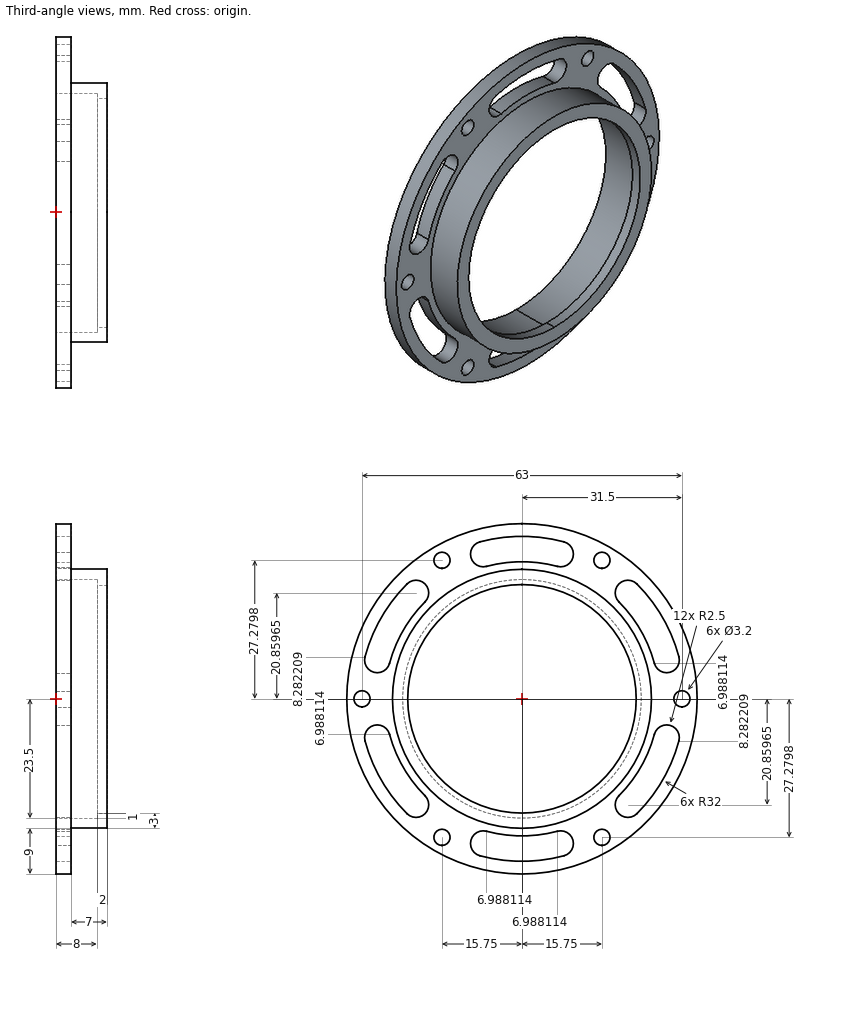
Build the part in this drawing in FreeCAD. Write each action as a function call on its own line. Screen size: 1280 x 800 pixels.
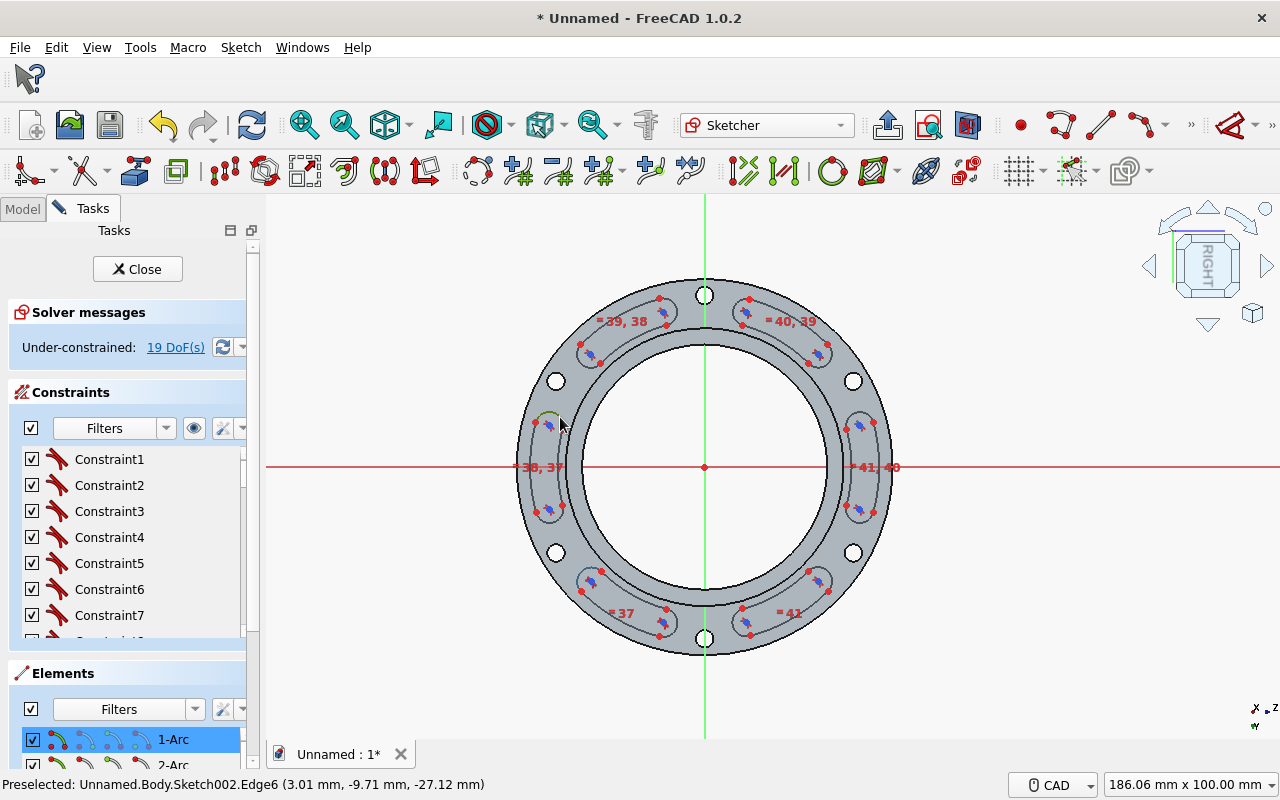
click(676, 317)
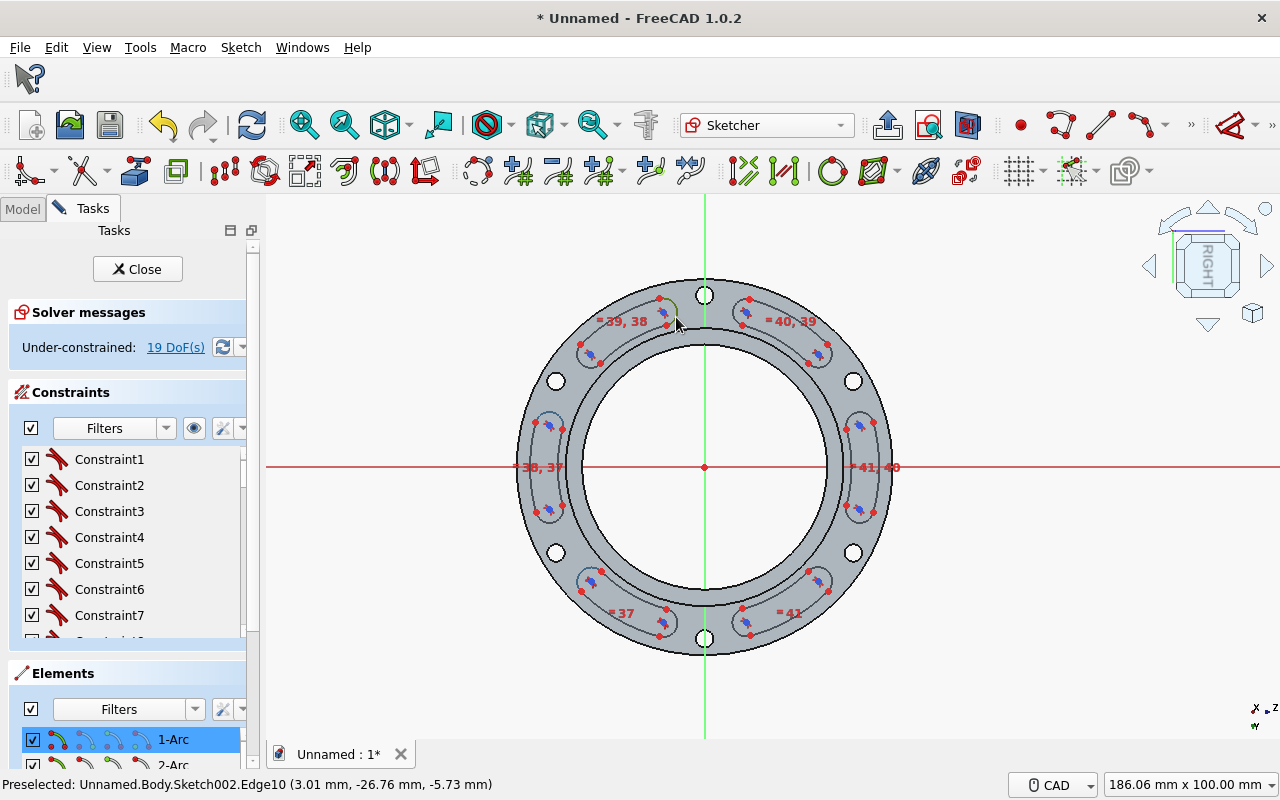
click(820, 367)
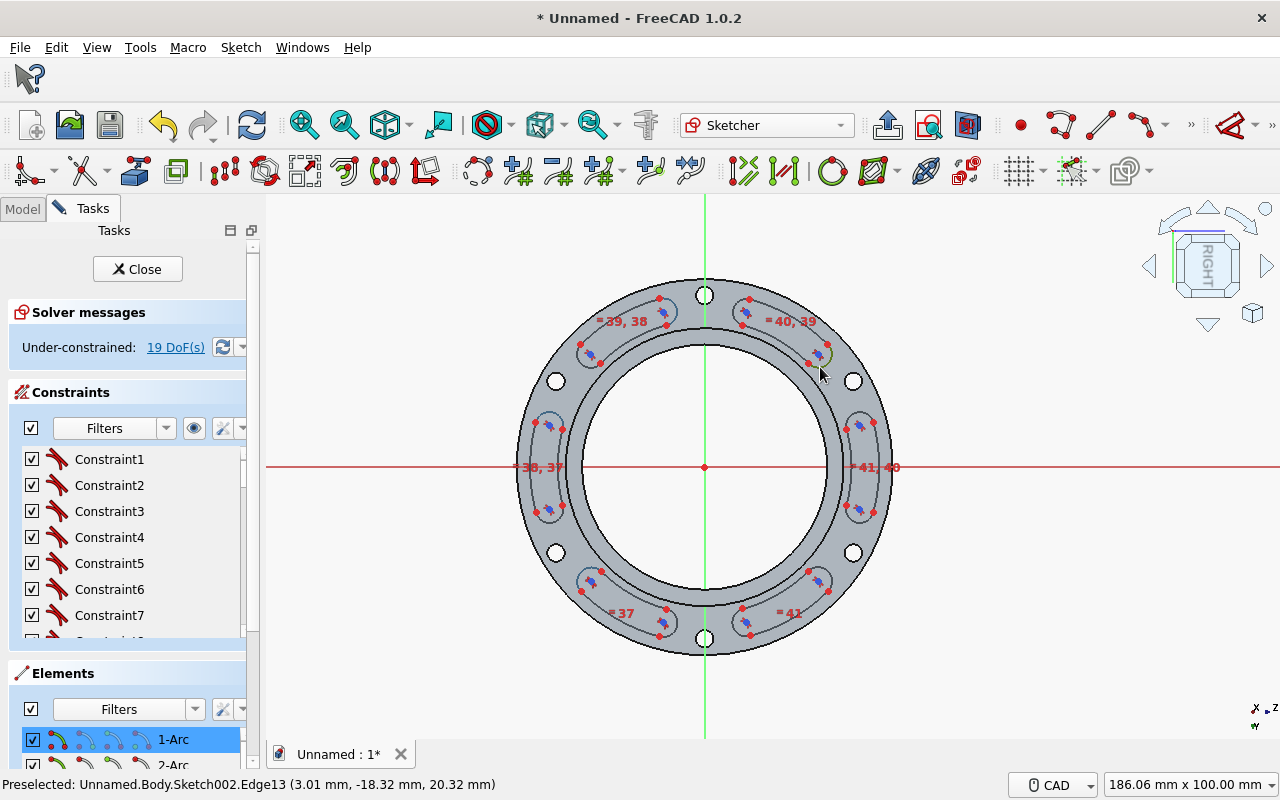
click(849, 518)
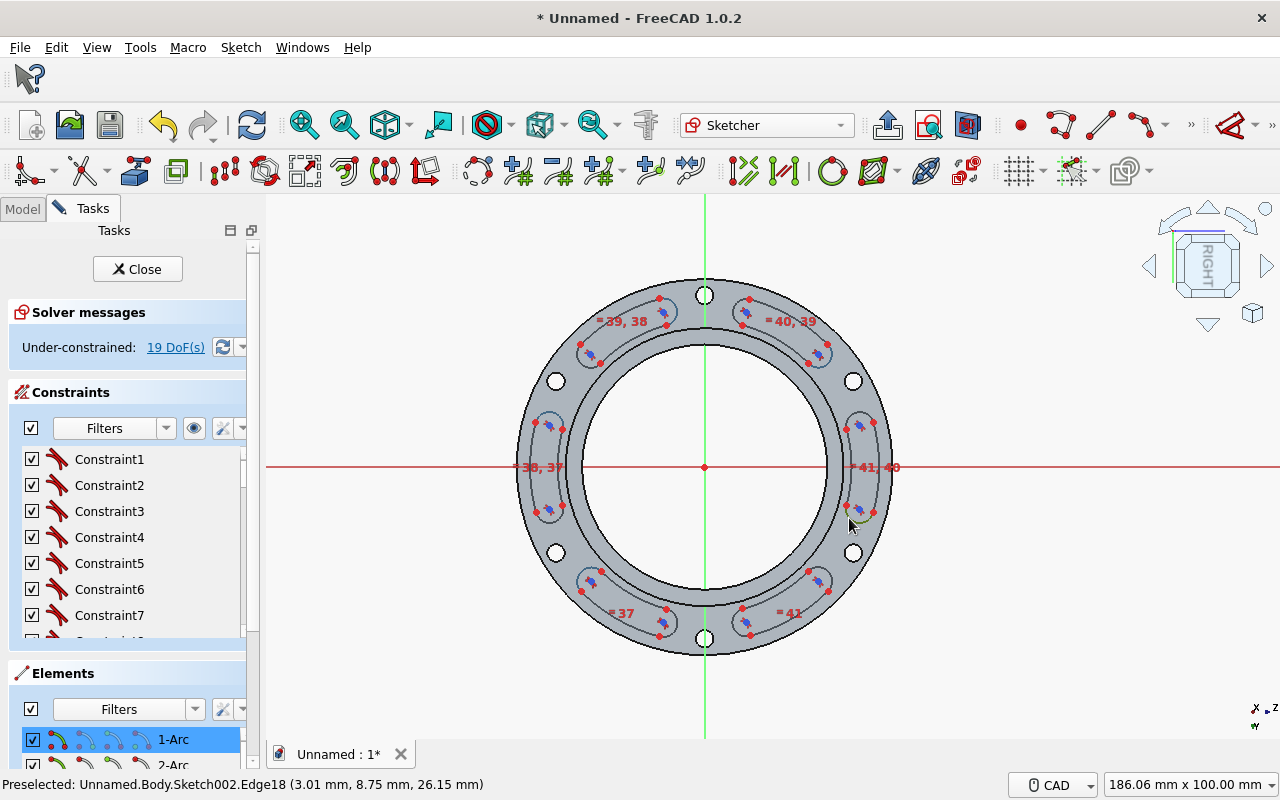
click(733, 617)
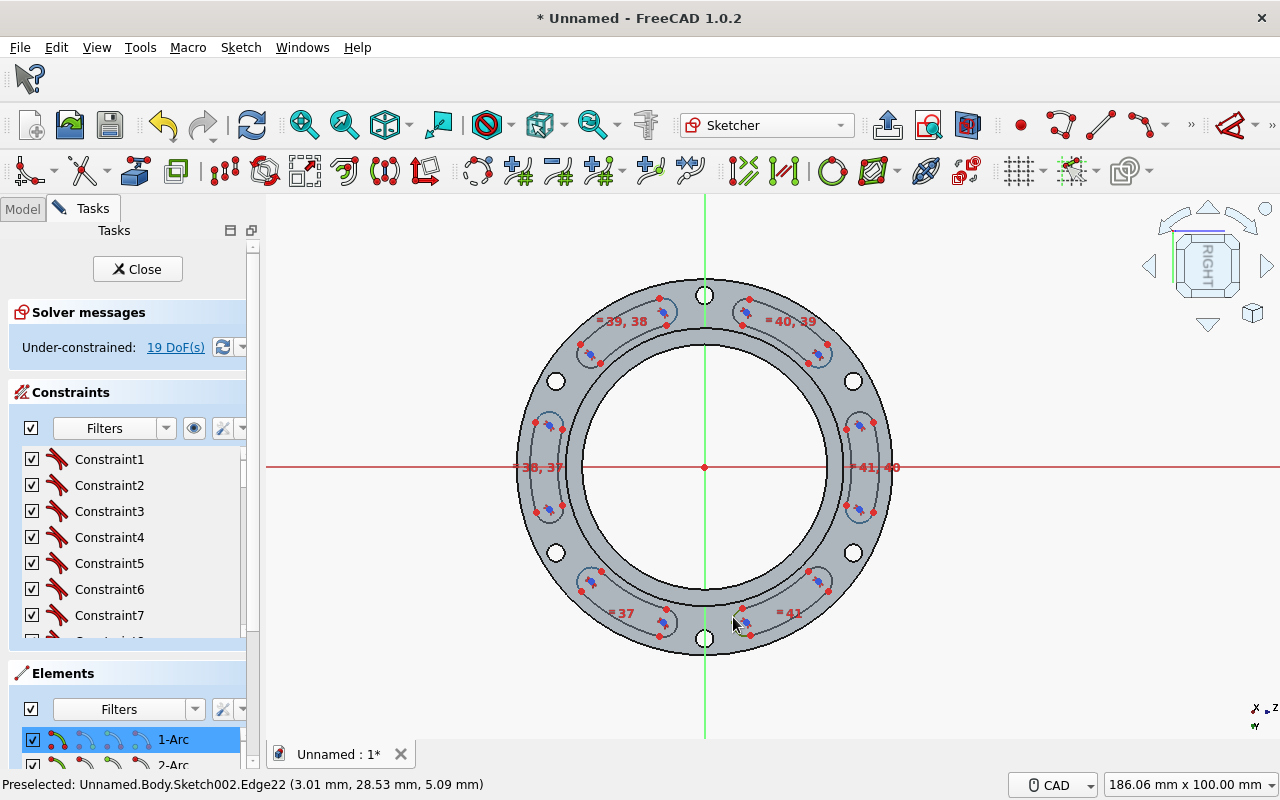
key(e)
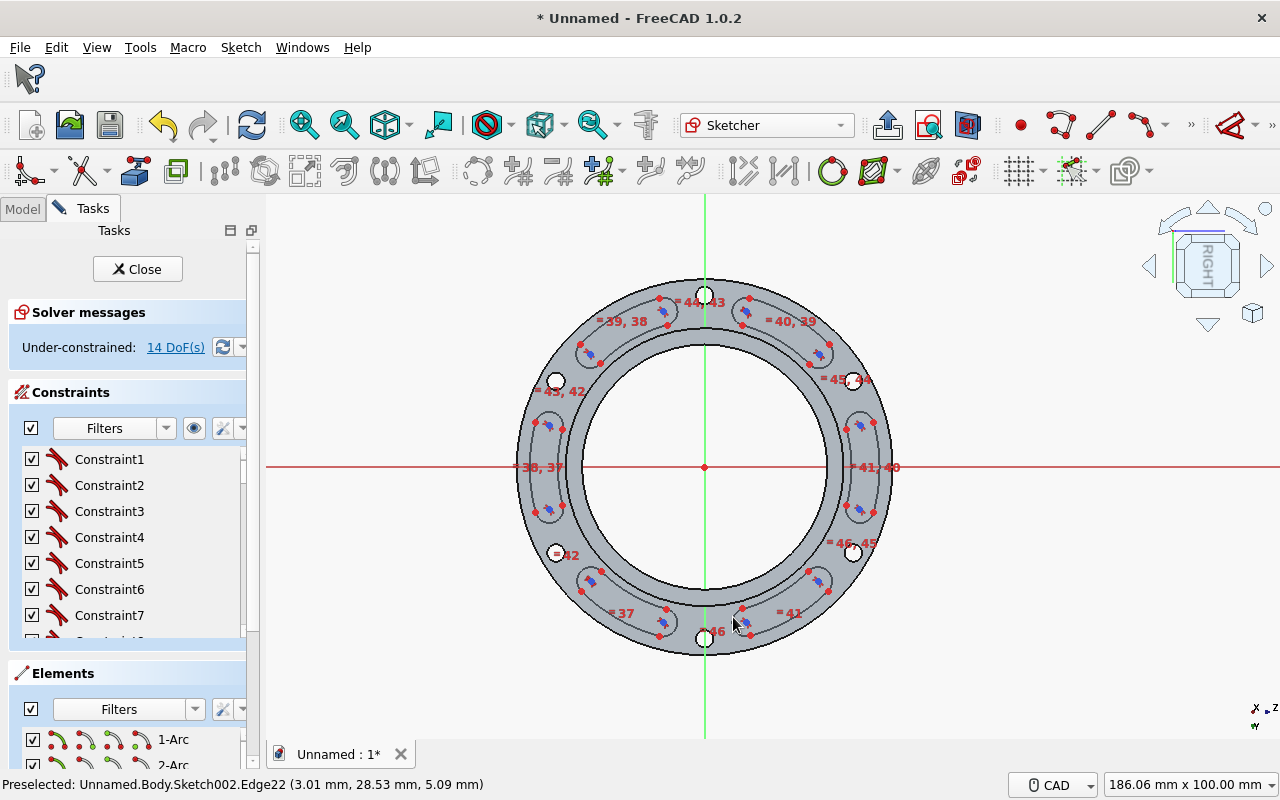
key(d)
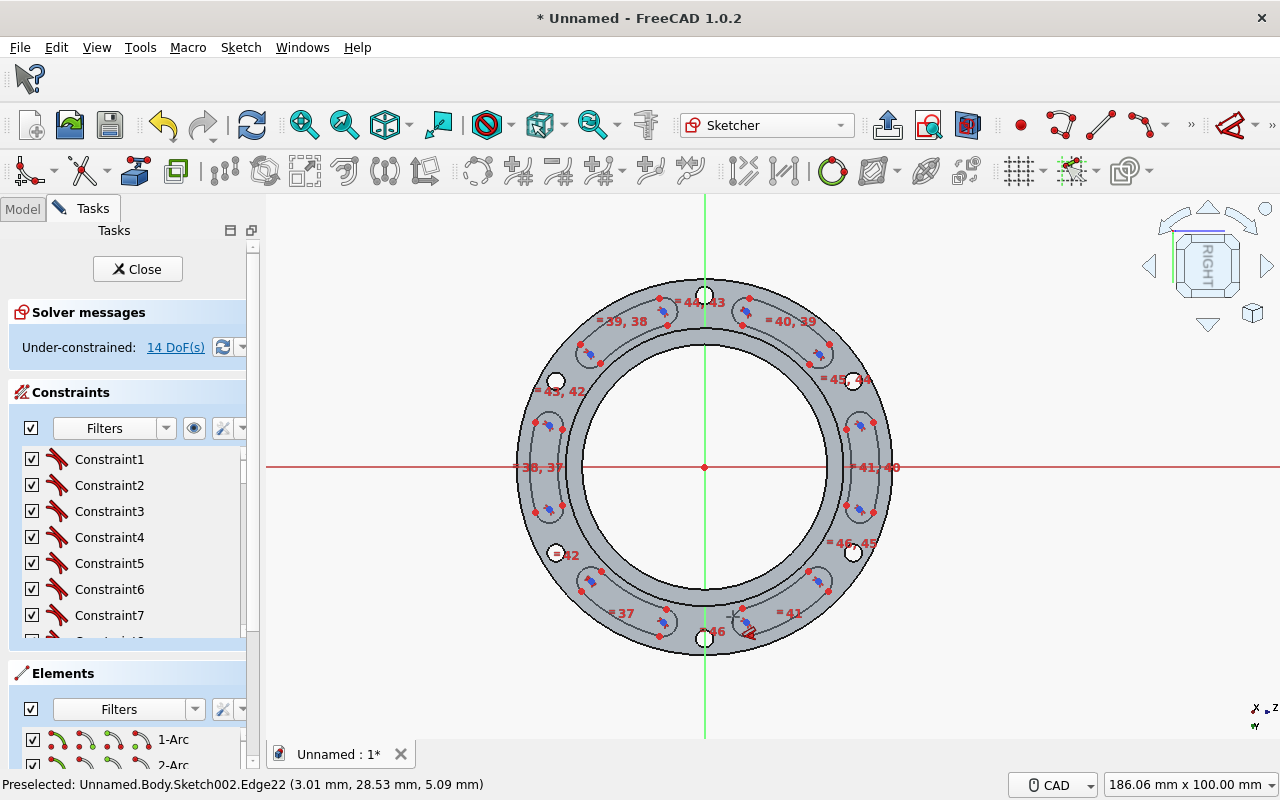
scroll(589, 567, up, 6)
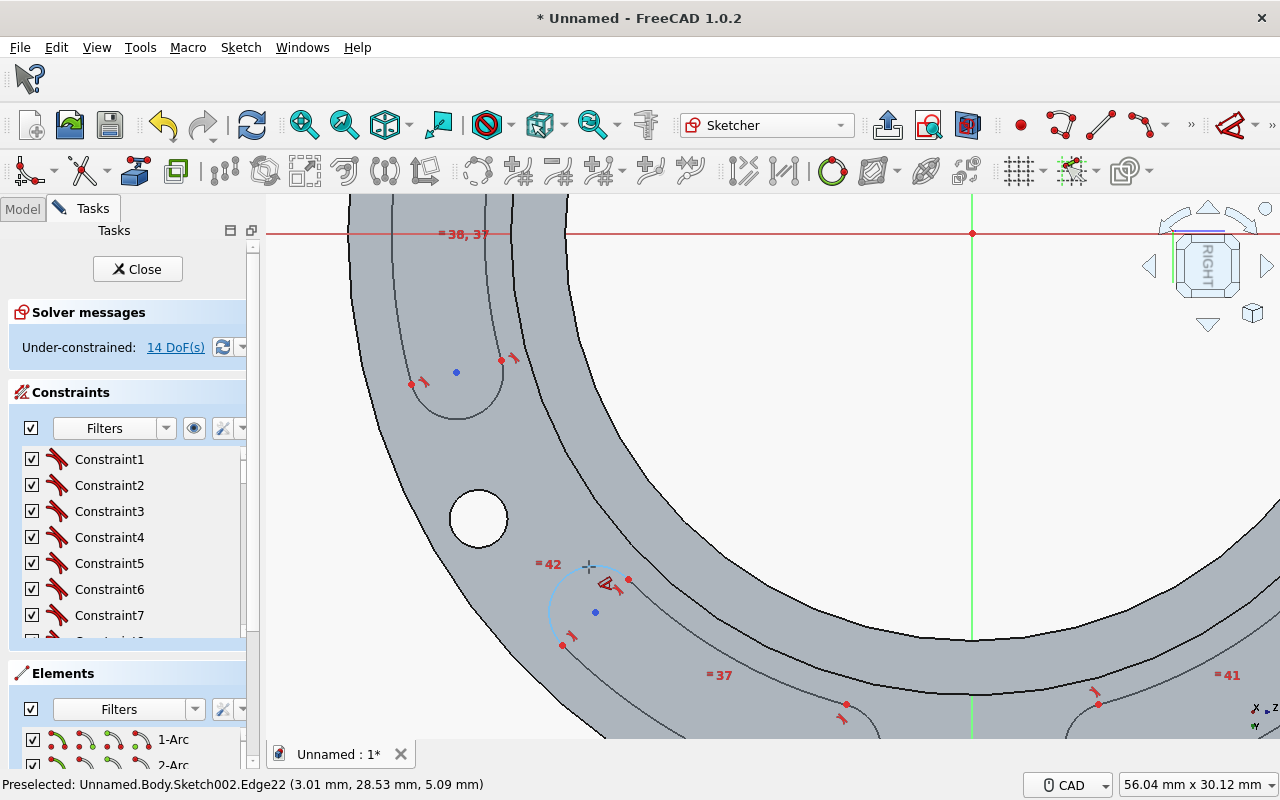
click(588, 566)
click(583, 534)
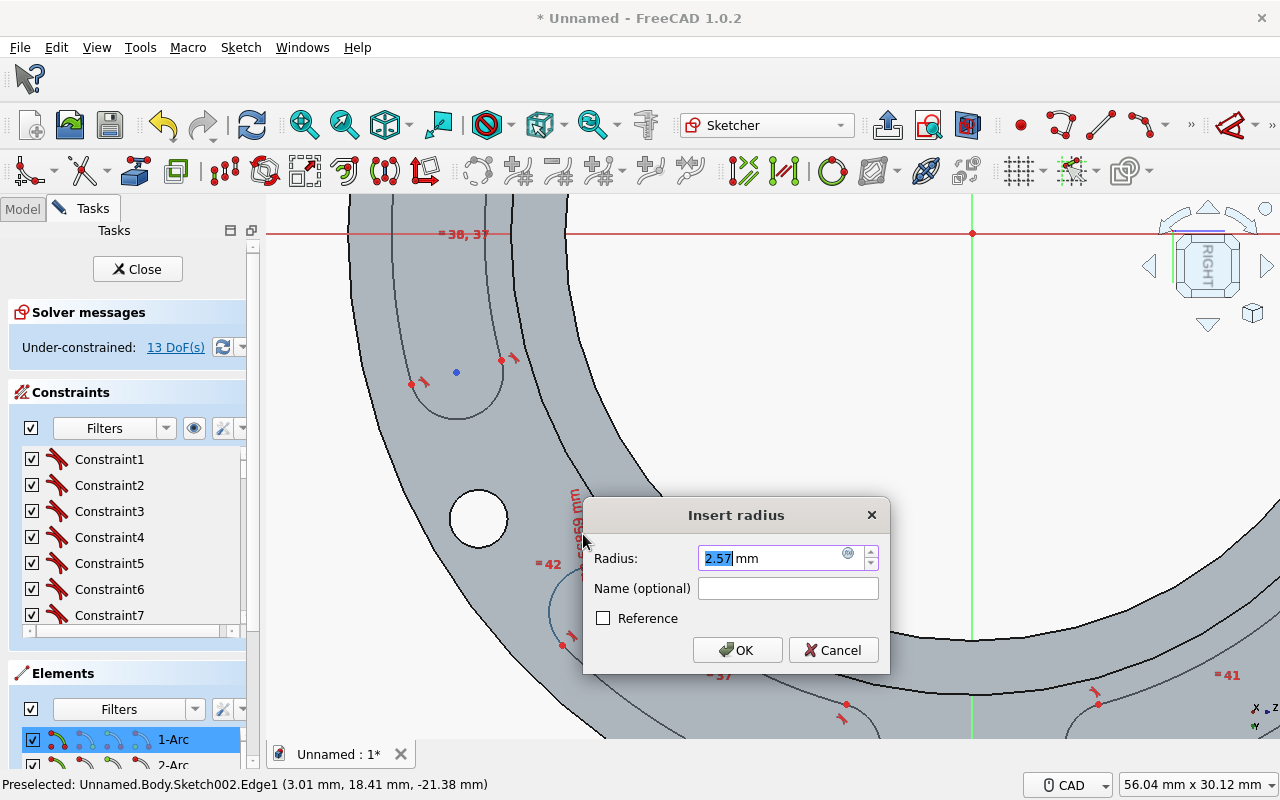
text(2.5)
key(Return)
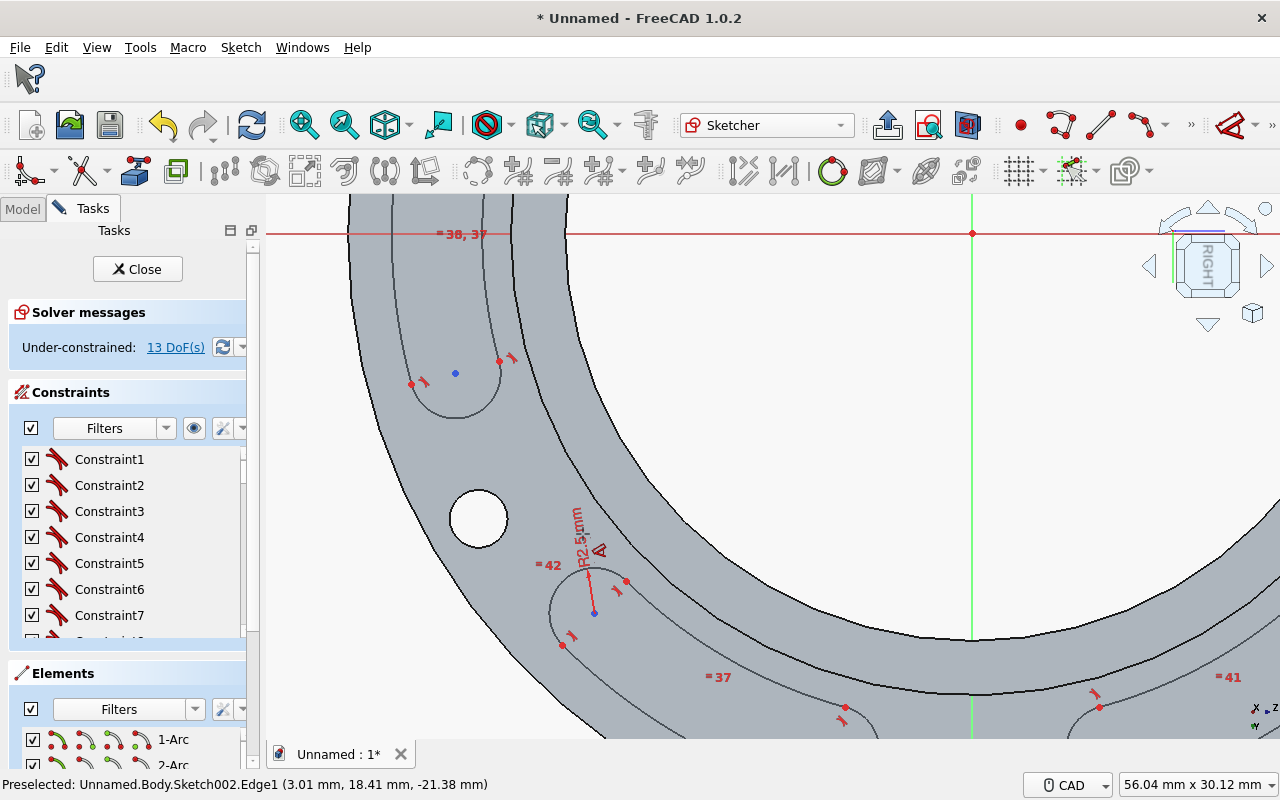
click(632, 704)
click(419, 497)